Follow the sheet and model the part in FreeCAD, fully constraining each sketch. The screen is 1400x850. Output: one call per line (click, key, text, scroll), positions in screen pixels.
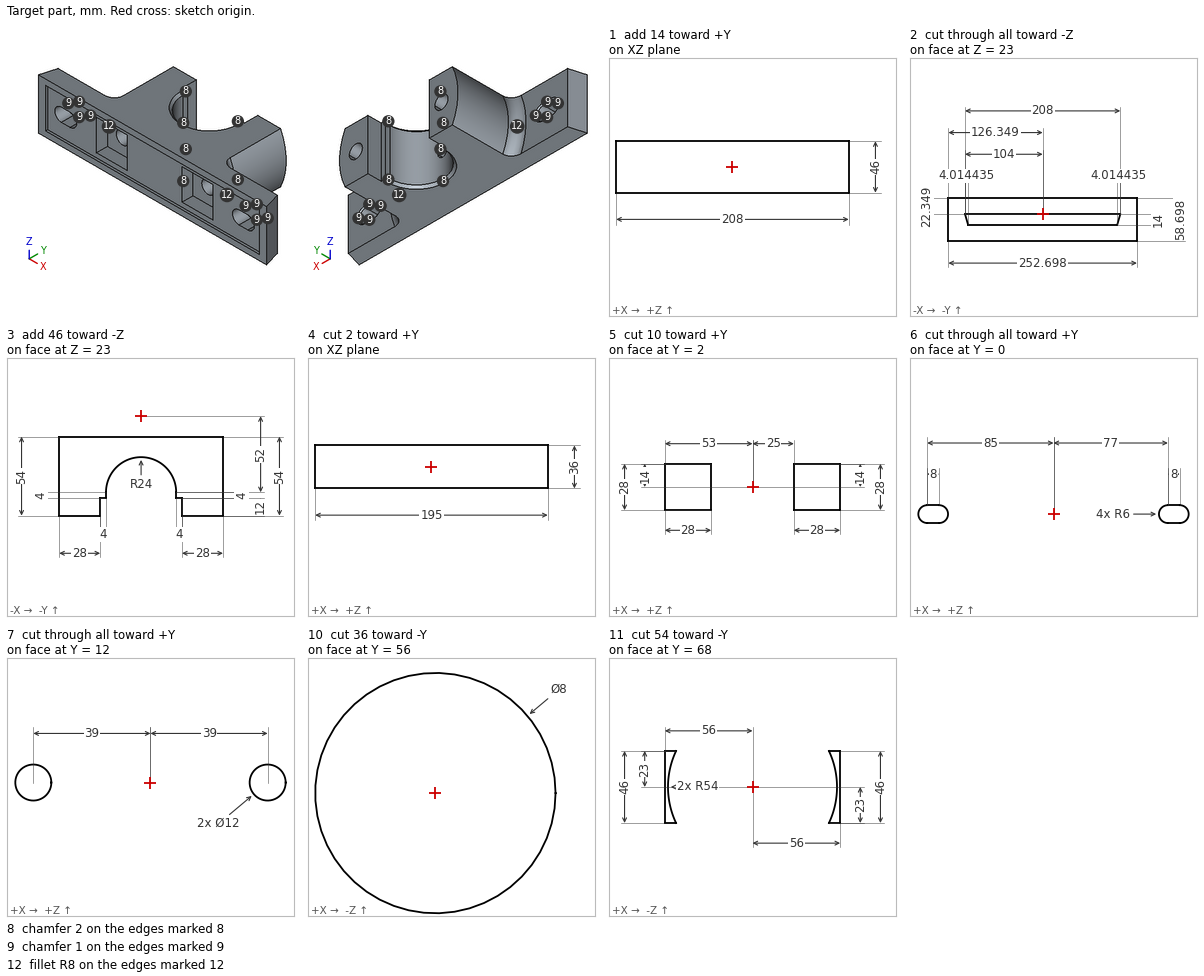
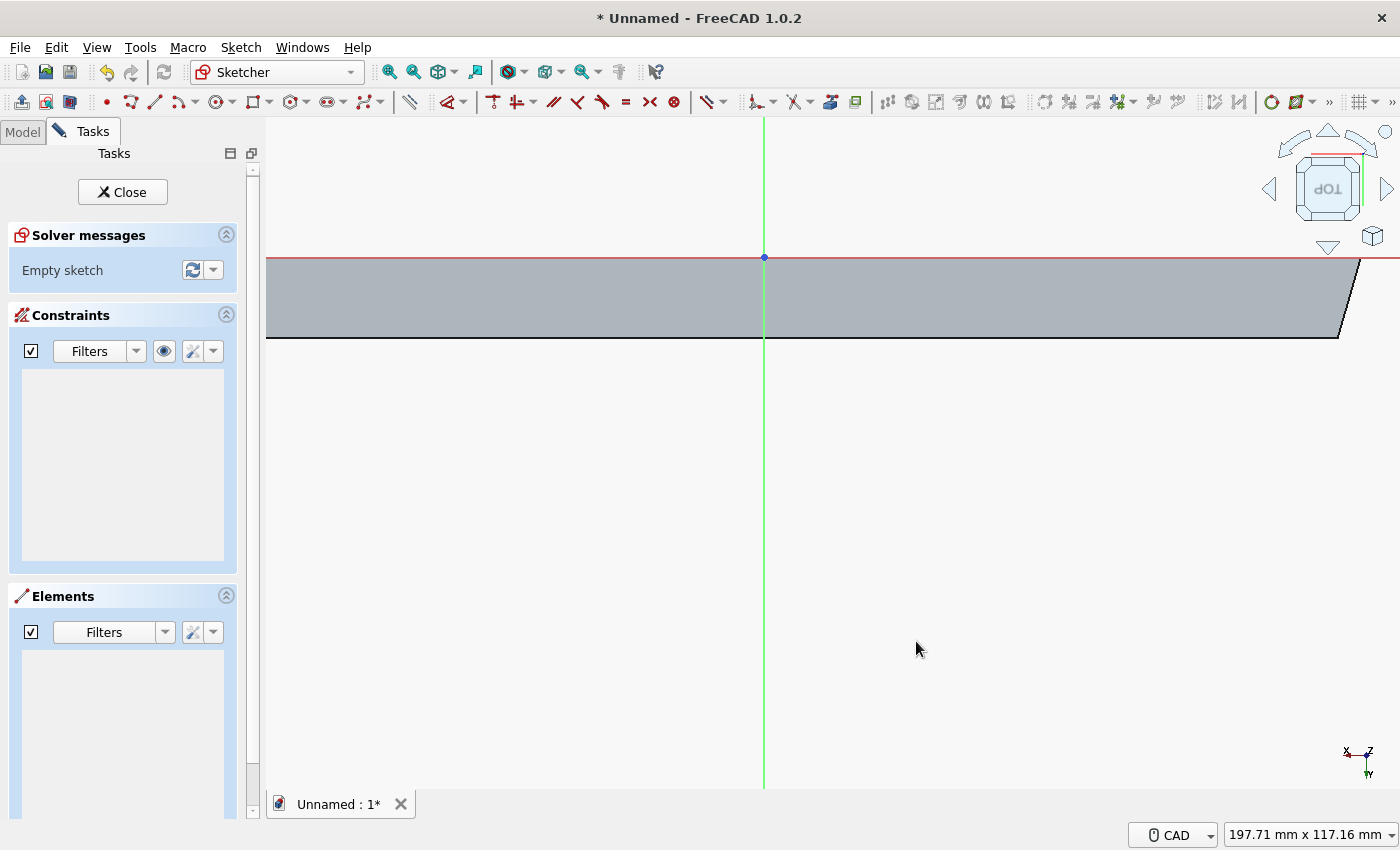
click(132, 102)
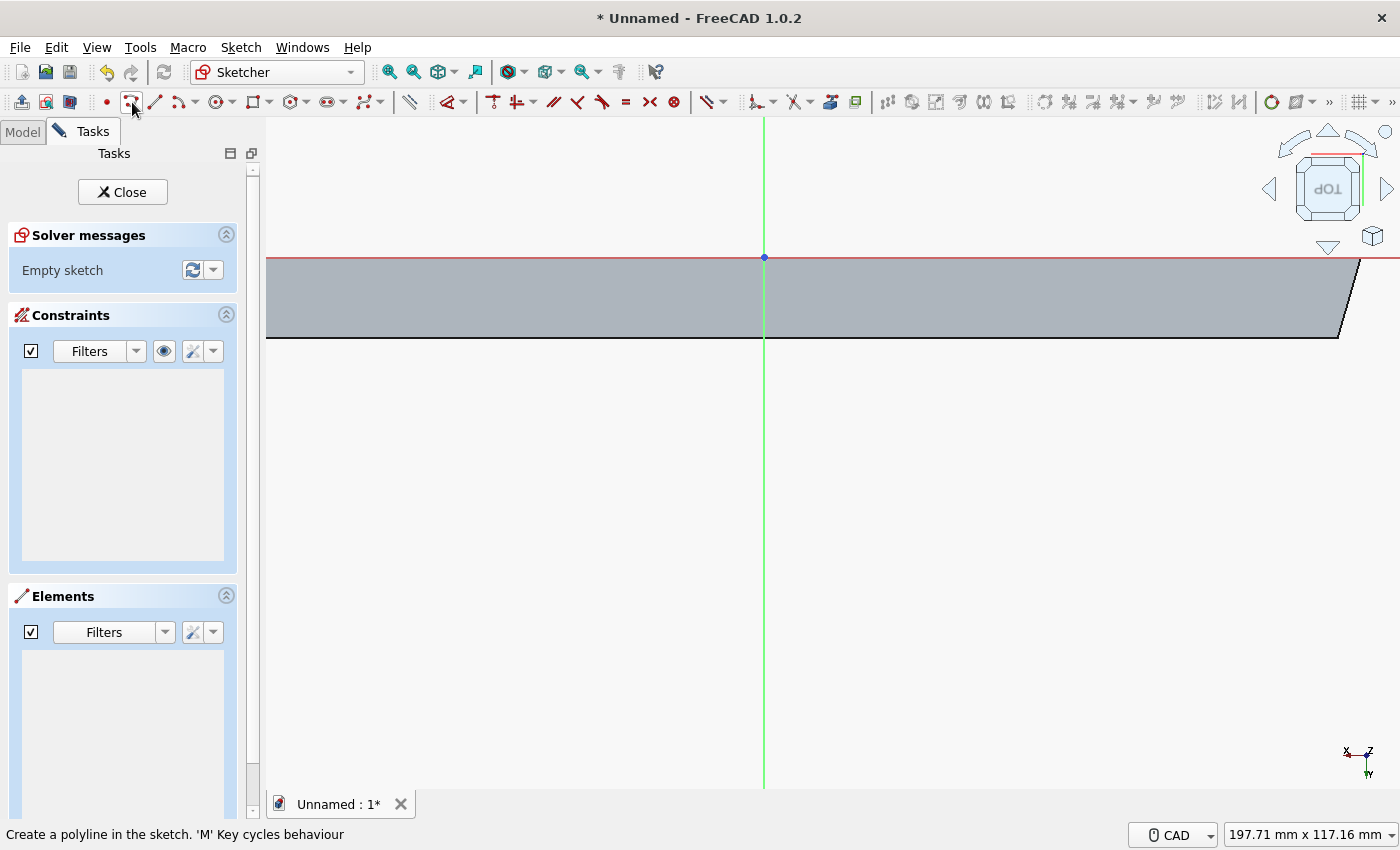
click(902, 556)
click(902, 579)
click(925, 579)
click(925, 648)
click(1085, 648)
click(1085, 338)
click(443, 338)
click(443, 648)
click(604, 648)
click(604, 579)
click(627, 579)
click(627, 556)
right_click(627, 556)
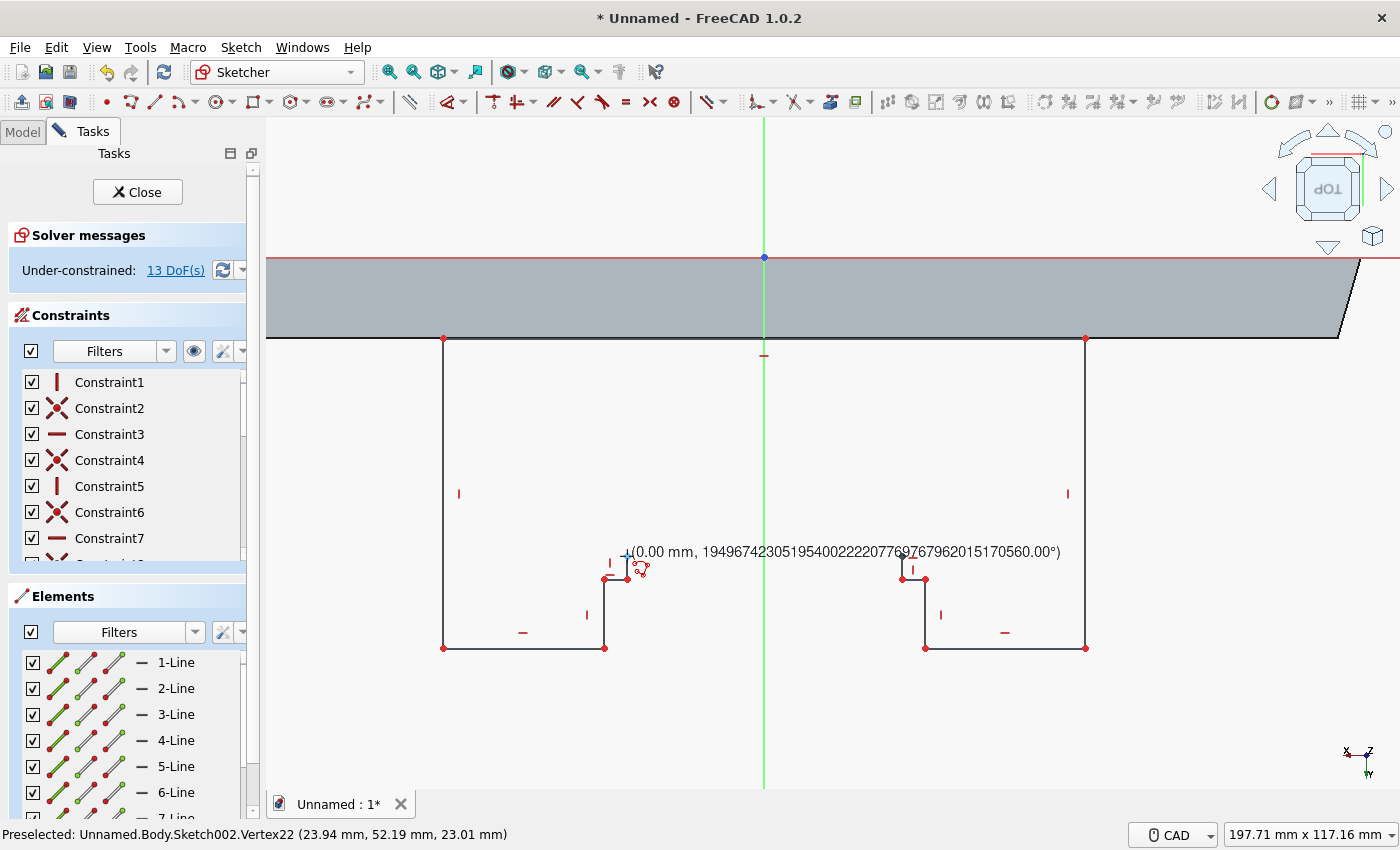
key(g)
key(3)
key(a)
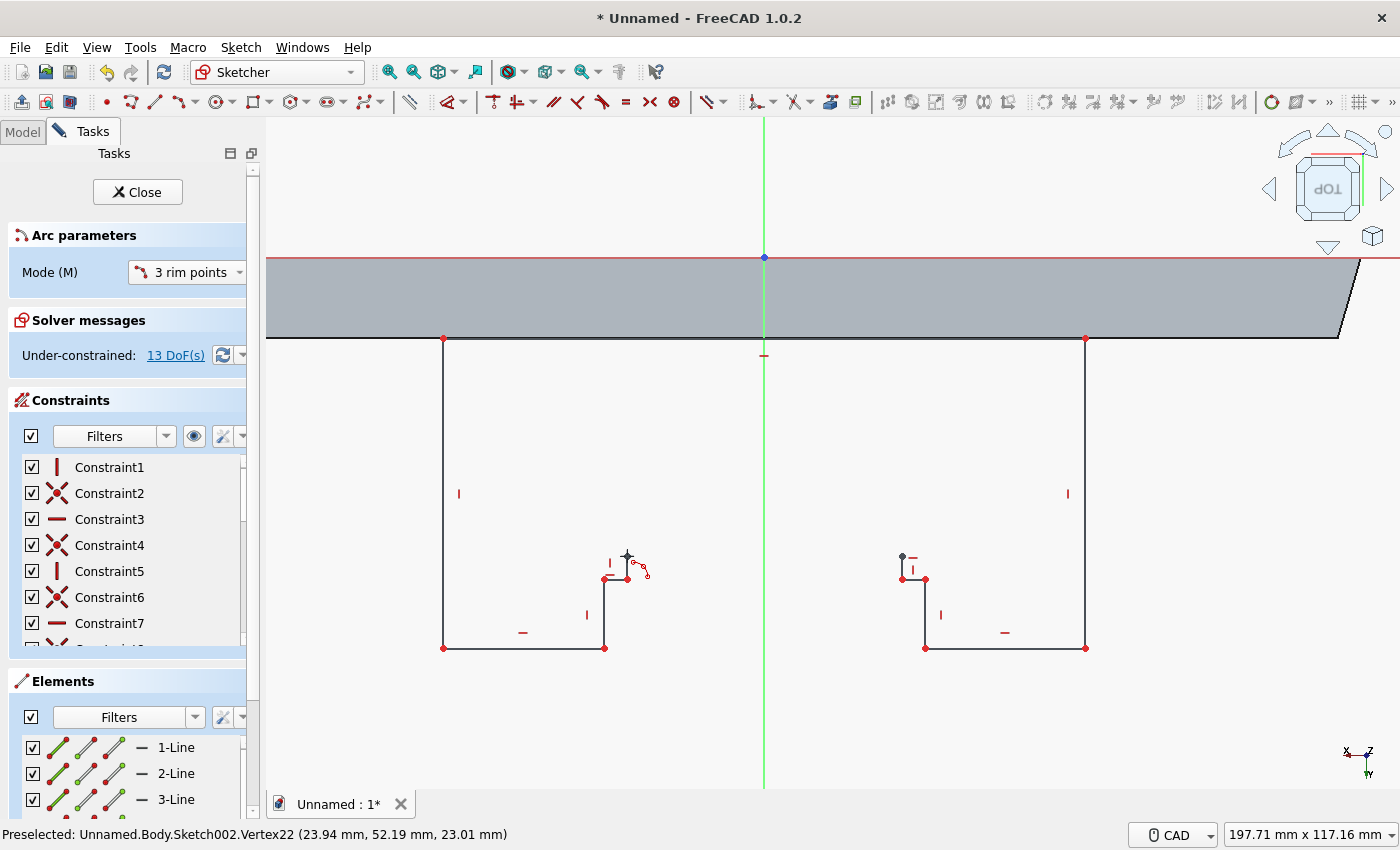
scroll(627, 556, up, 2)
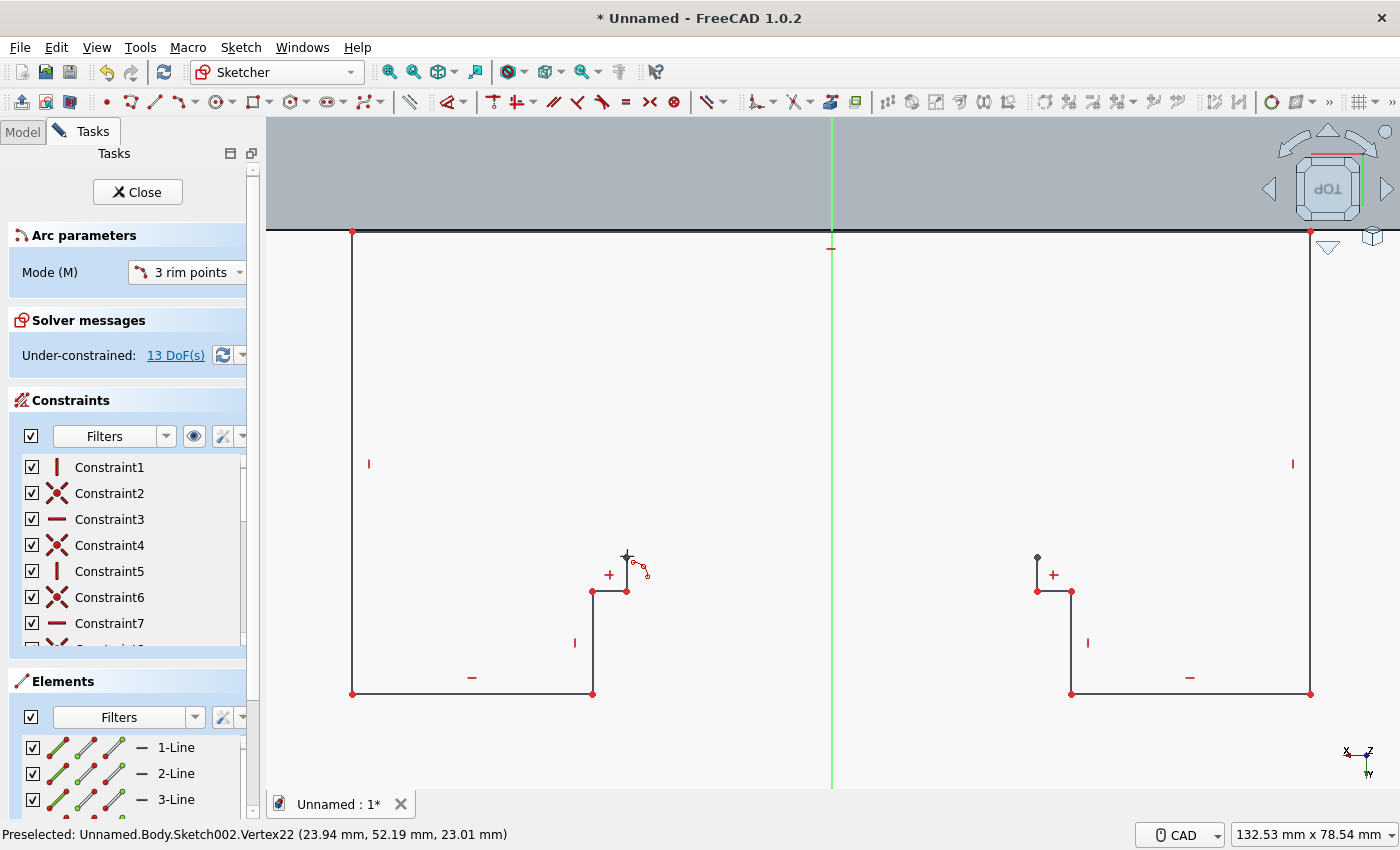
click(627, 557)
click(1037, 557)
click(895, 360)
key(Escape)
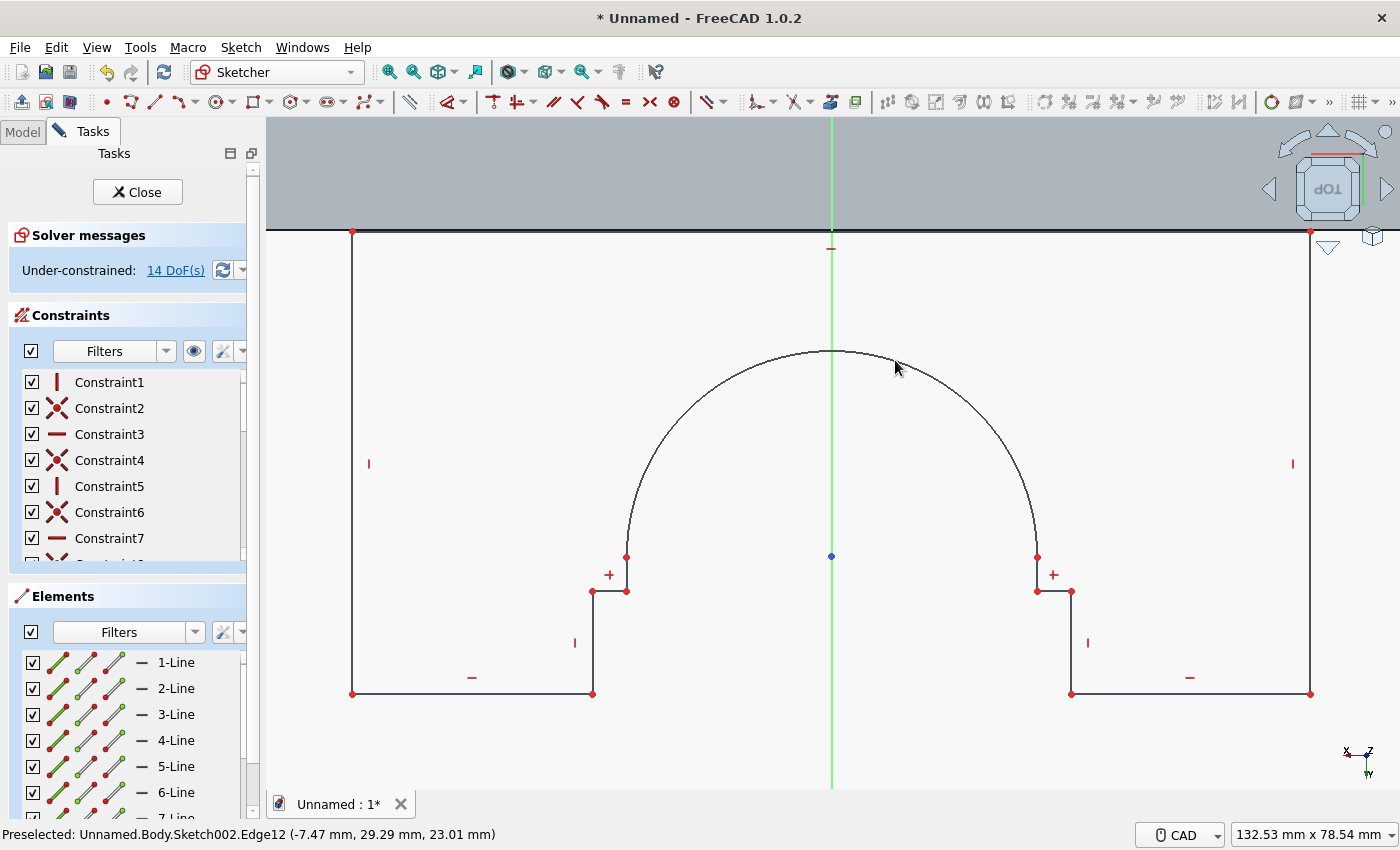
scroll(1037, 567, up, 2)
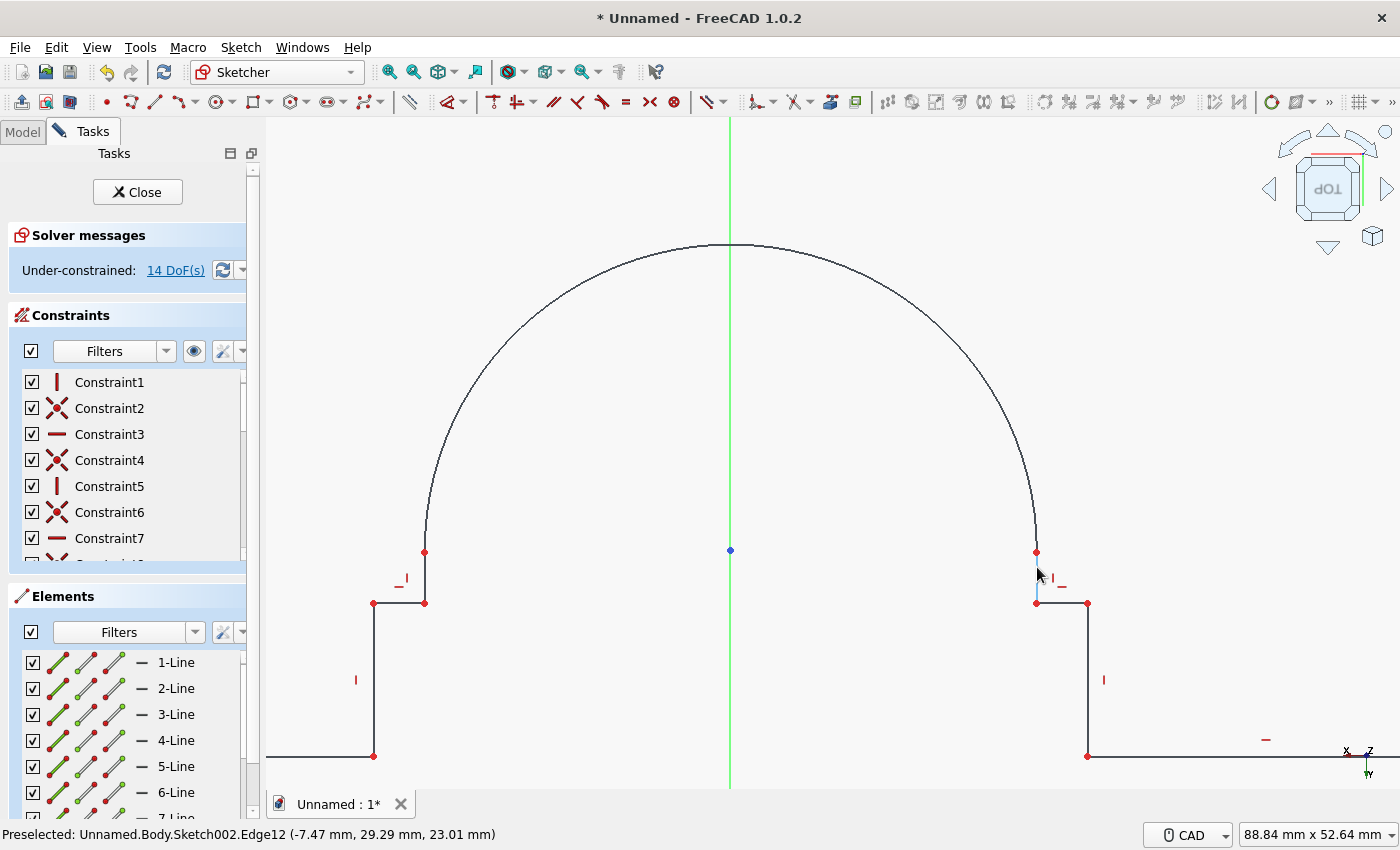
click(1037, 567)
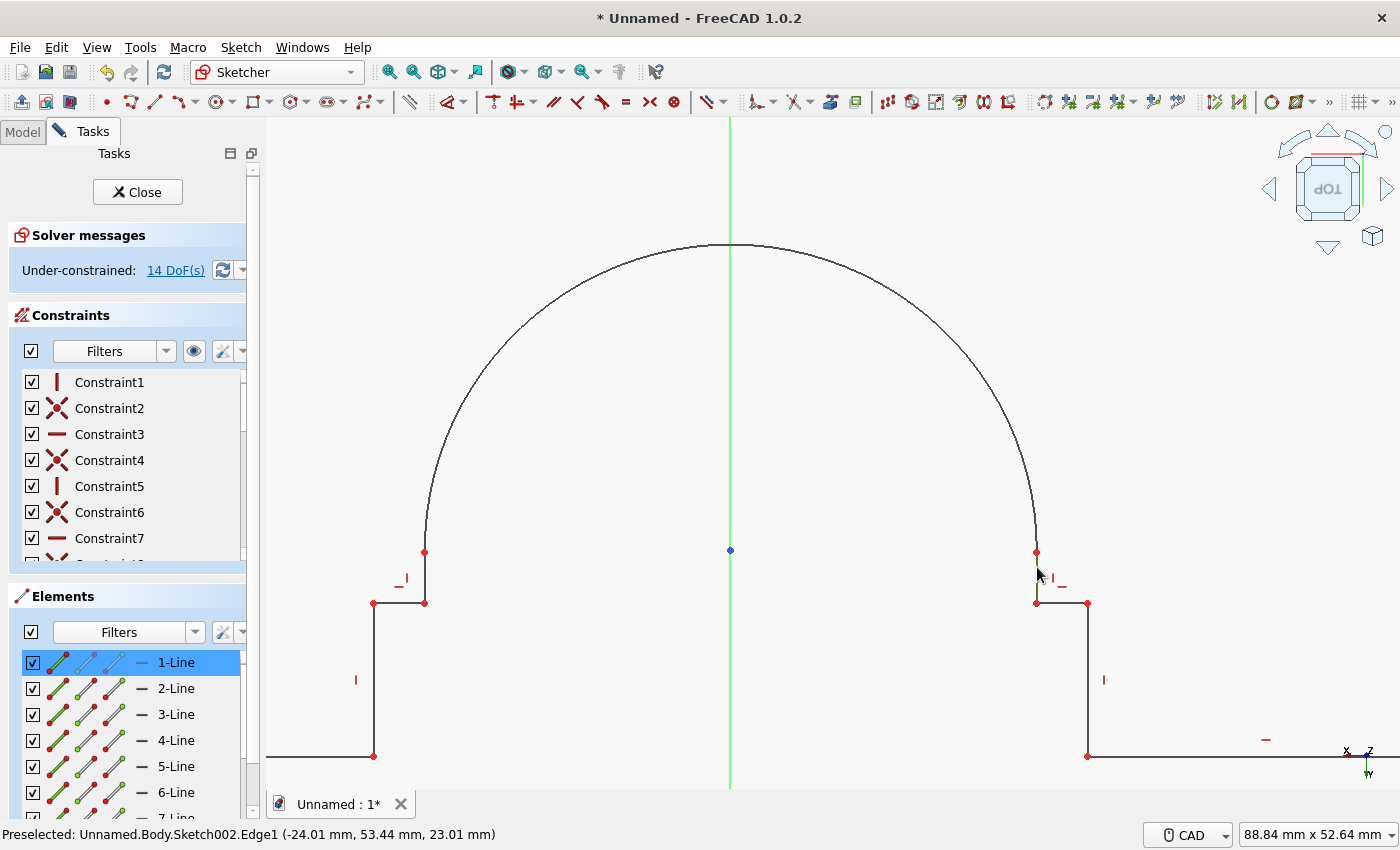
click(911, 303)